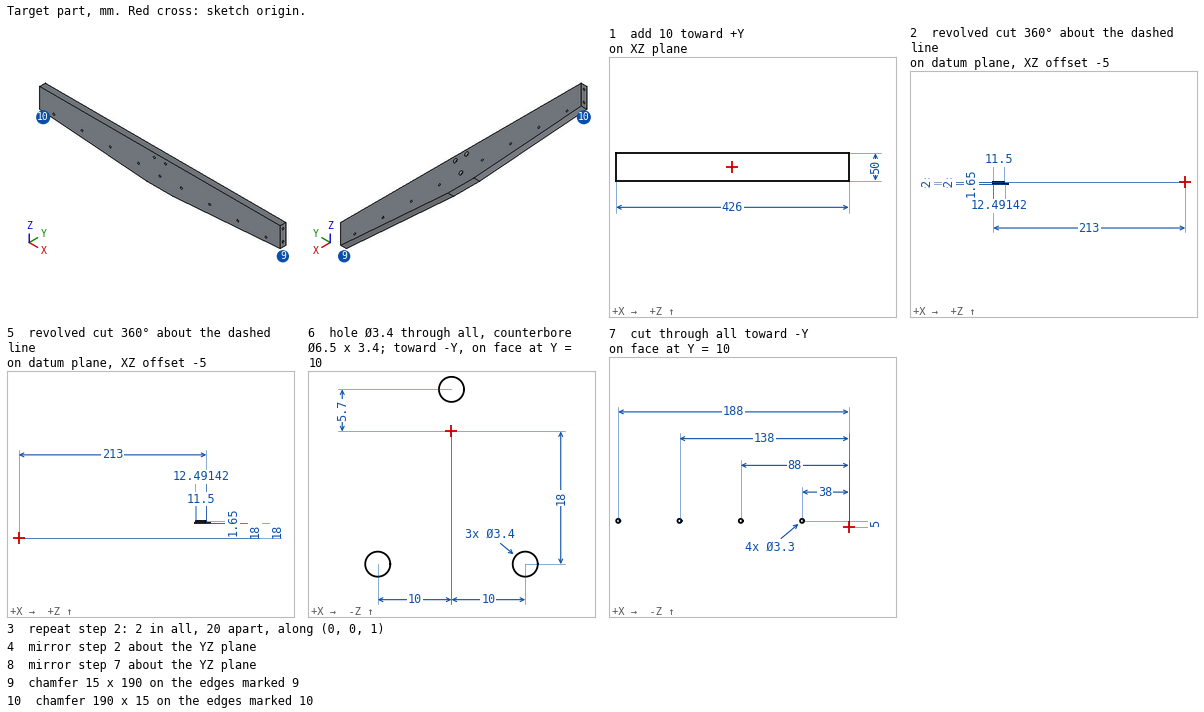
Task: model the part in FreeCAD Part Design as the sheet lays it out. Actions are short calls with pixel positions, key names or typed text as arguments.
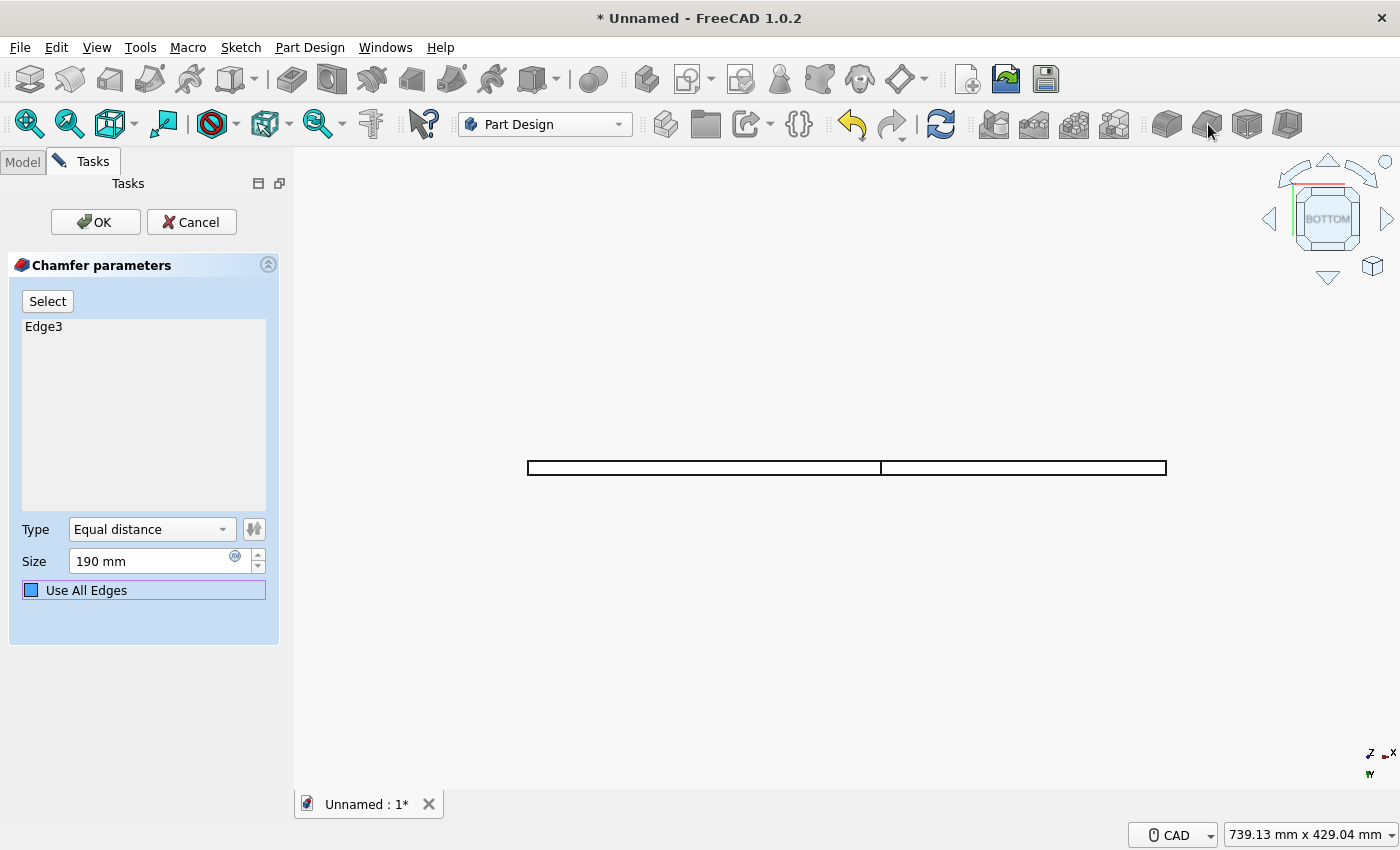
click(153, 530)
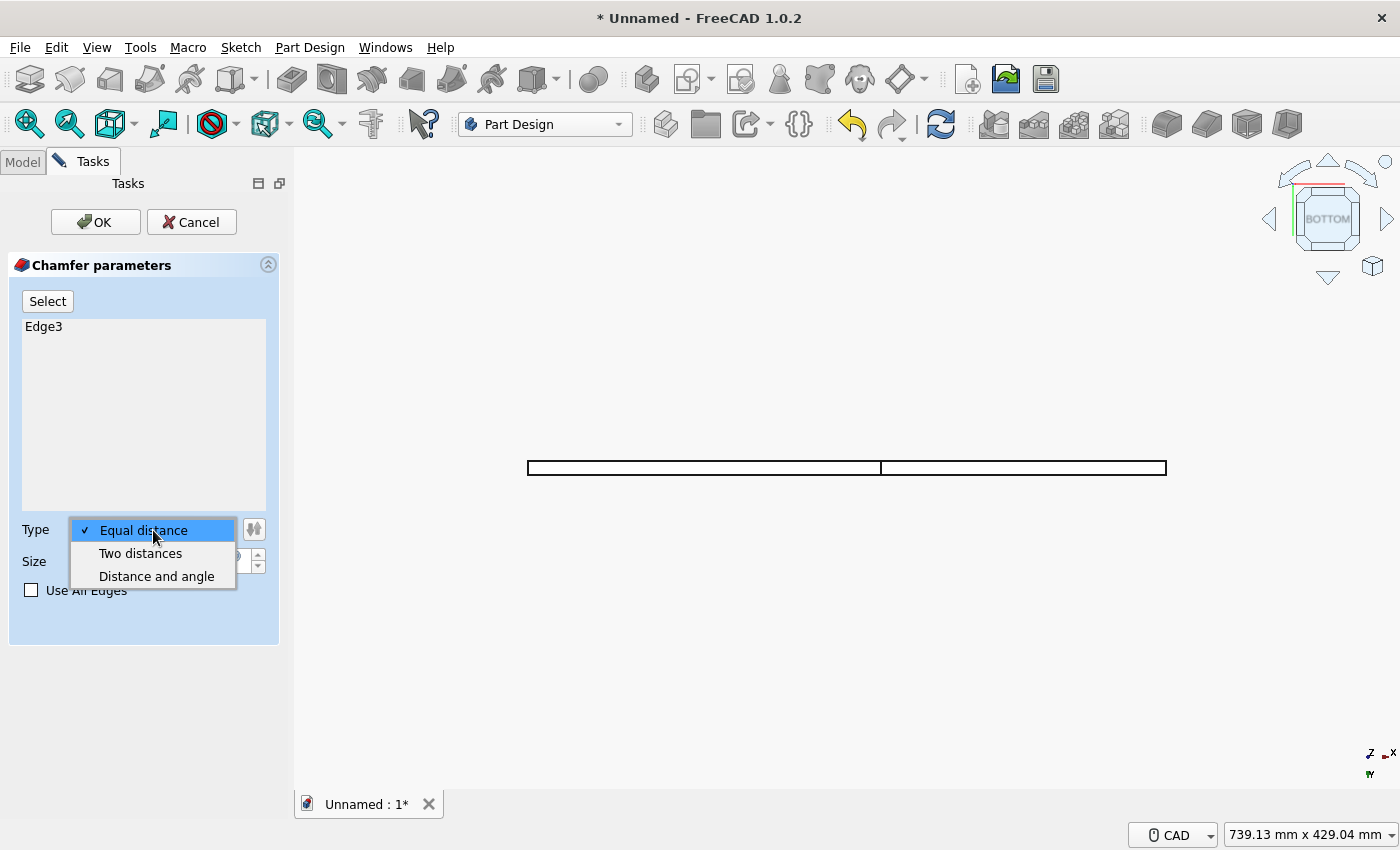
click(152, 554)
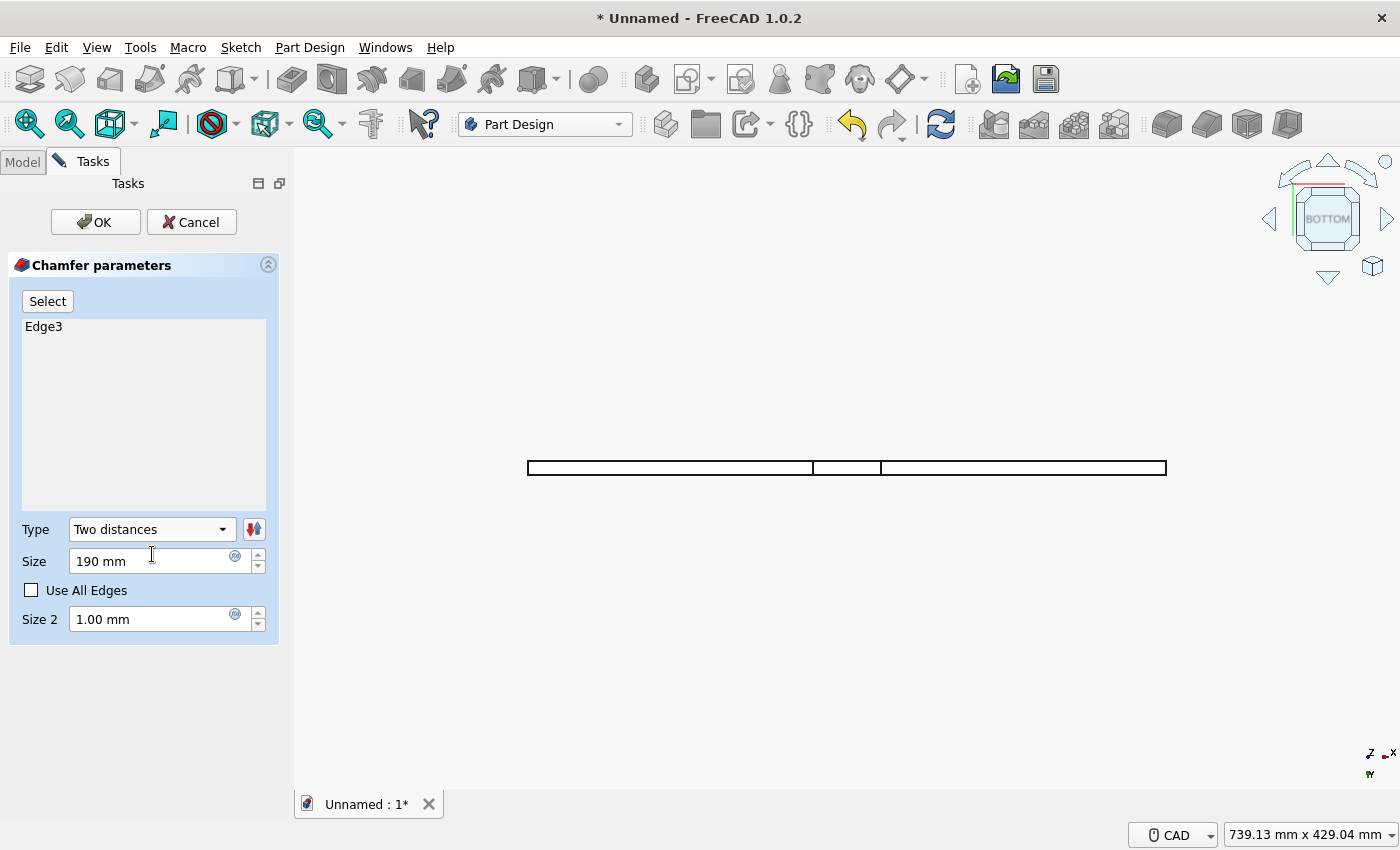
triple_click(160, 619)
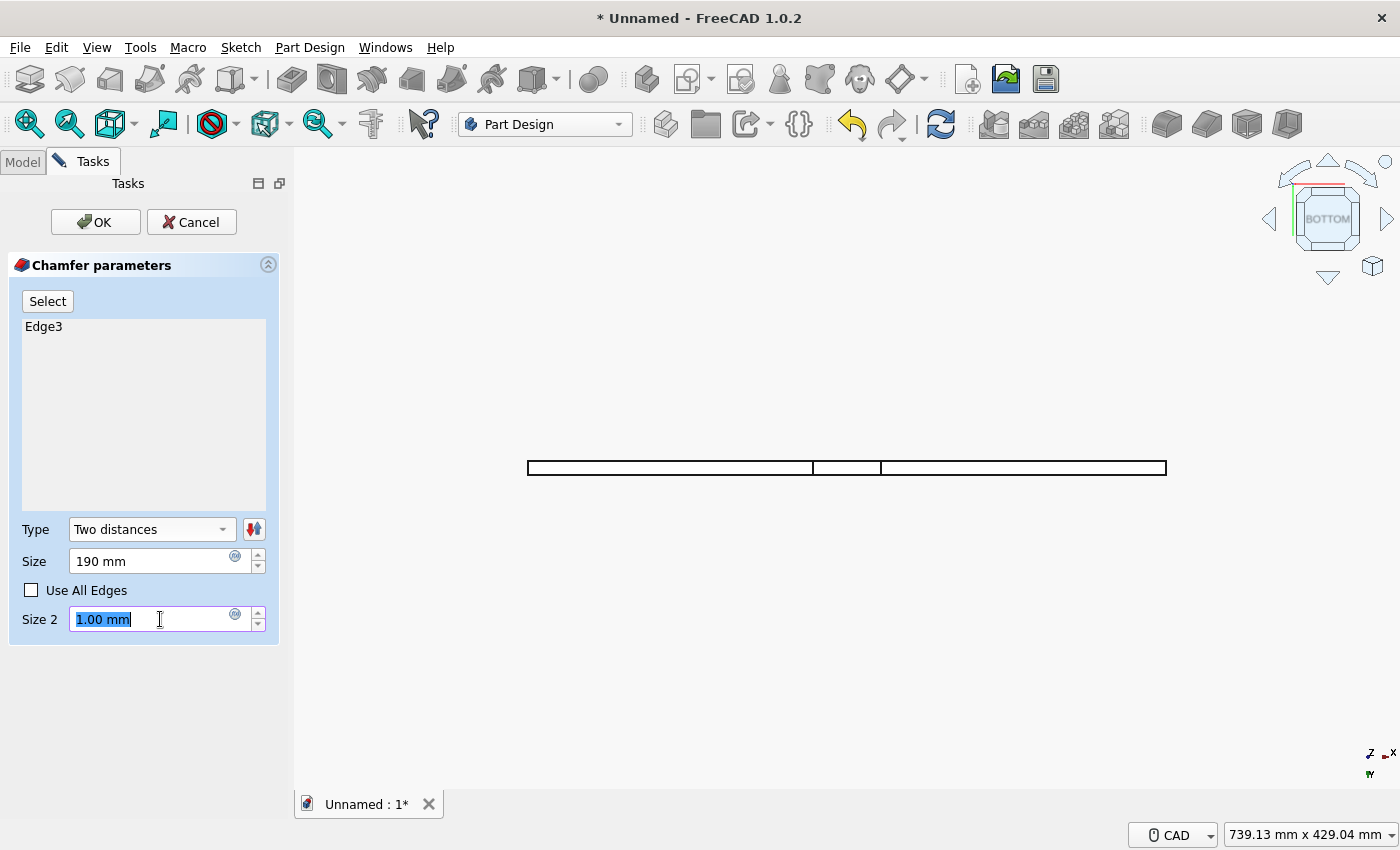
text(15)
key(Tab)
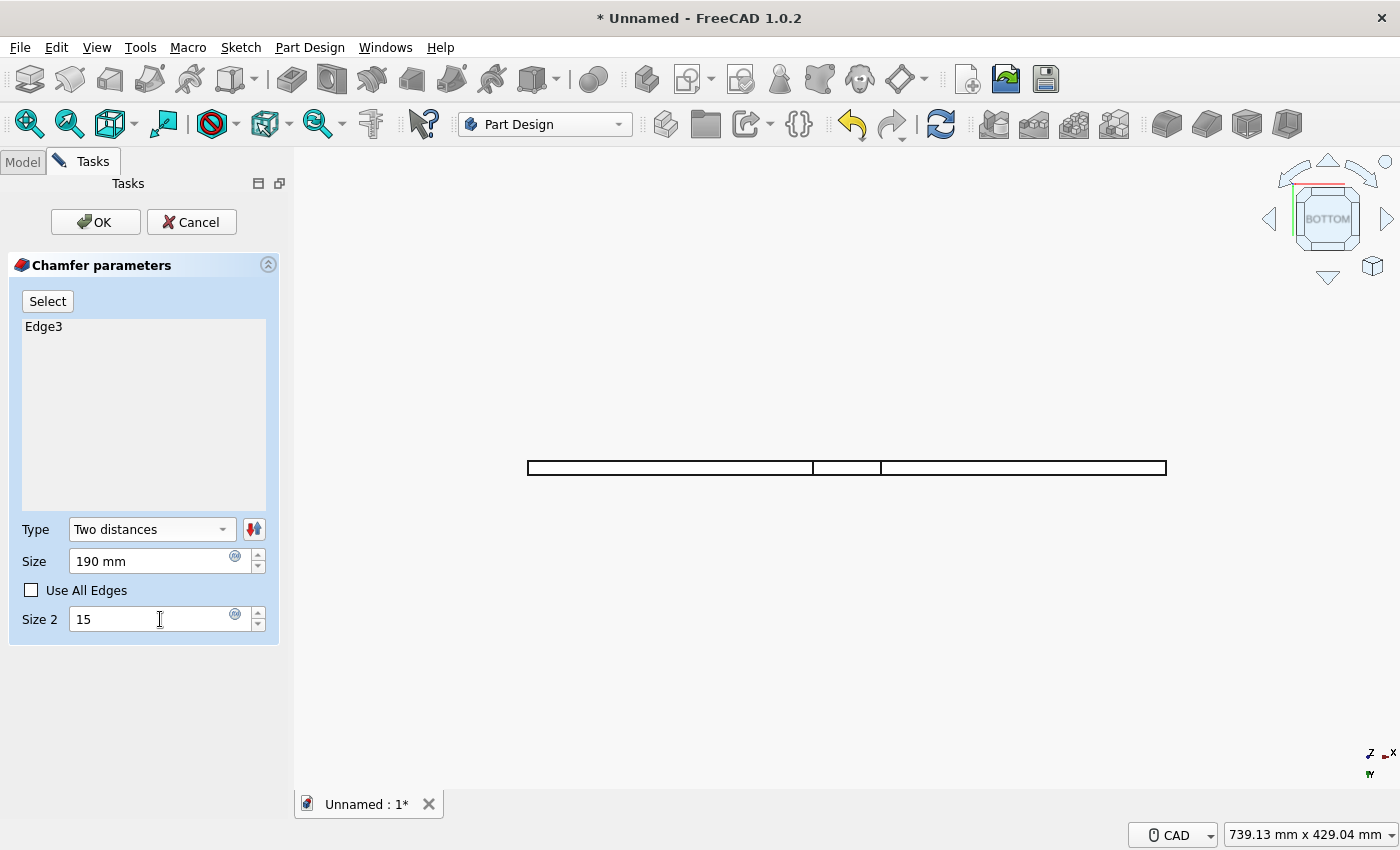
click(96, 222)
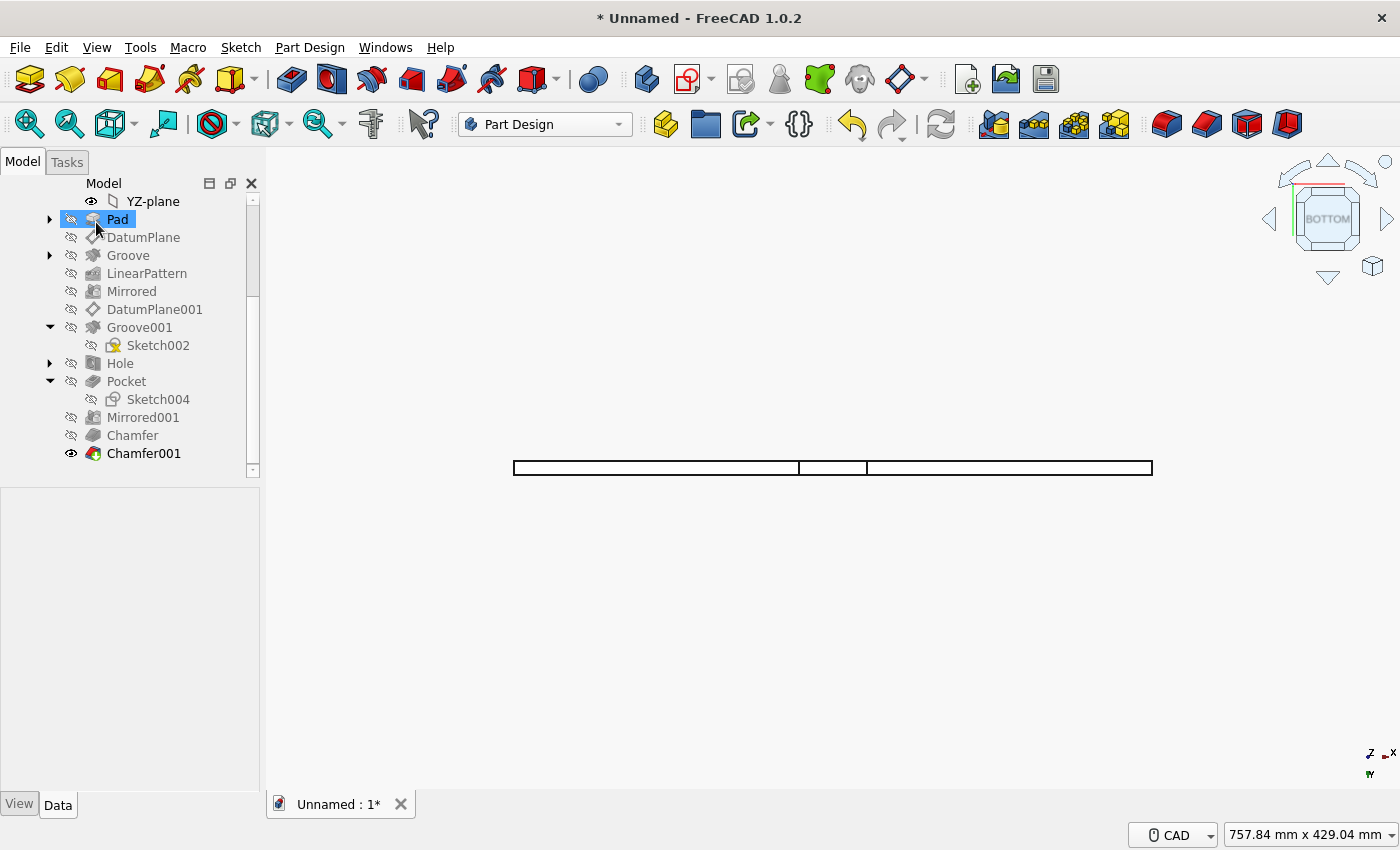
key(0)